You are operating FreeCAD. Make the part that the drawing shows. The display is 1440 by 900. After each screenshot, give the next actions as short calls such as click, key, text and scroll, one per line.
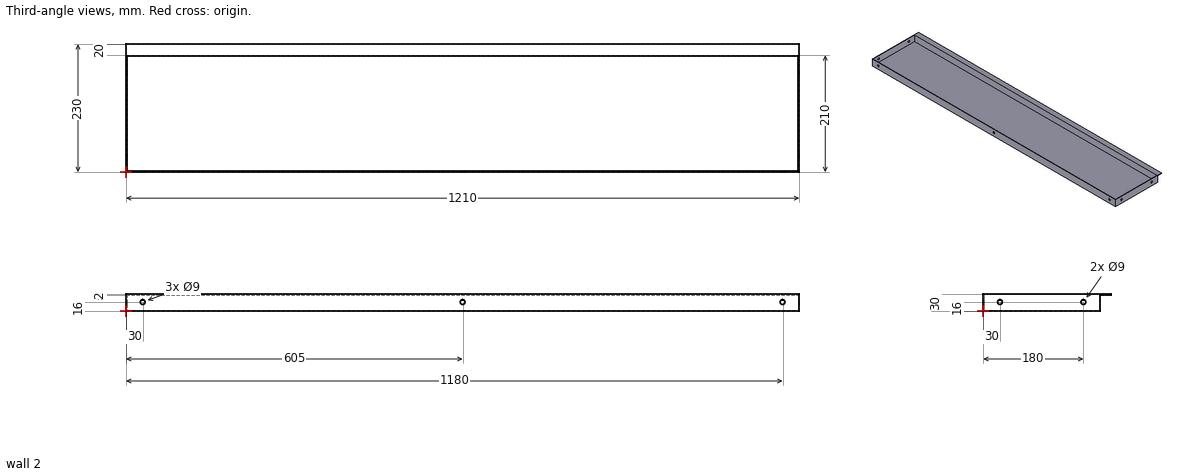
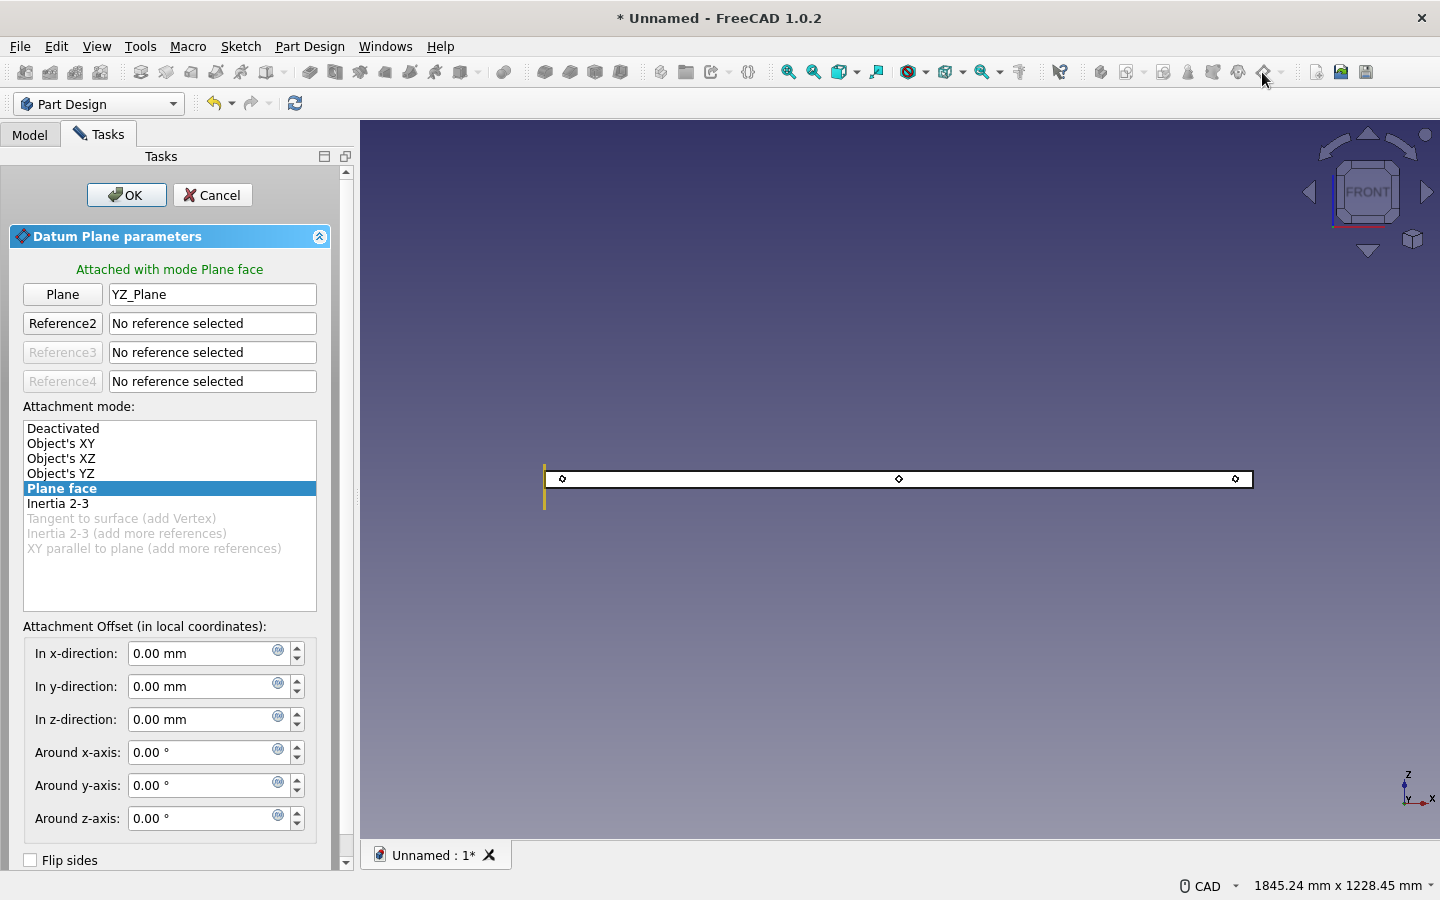
triple_click(210, 720)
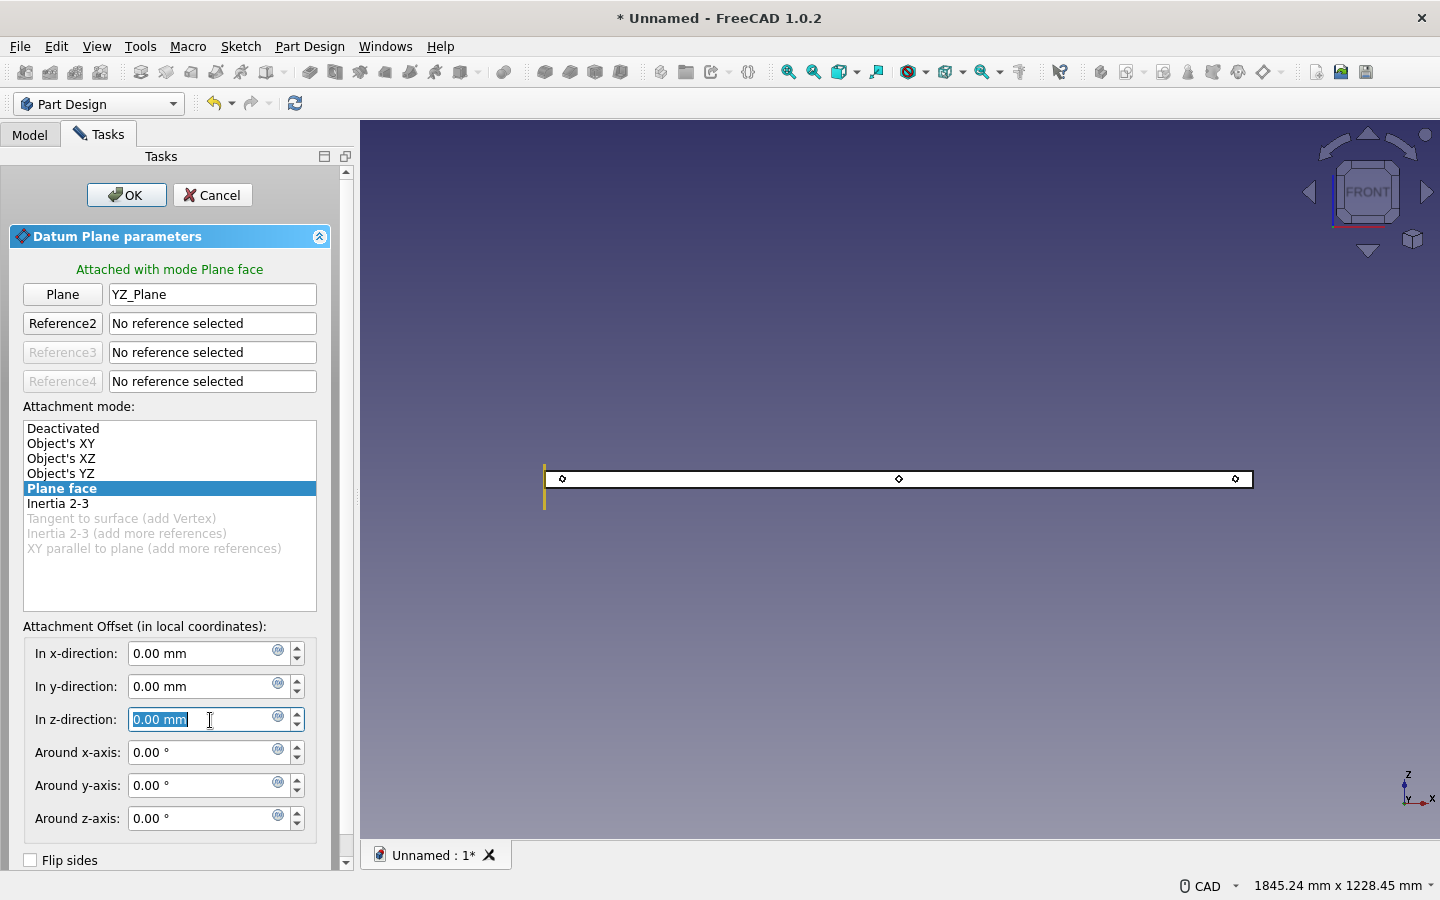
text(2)
key(Tab)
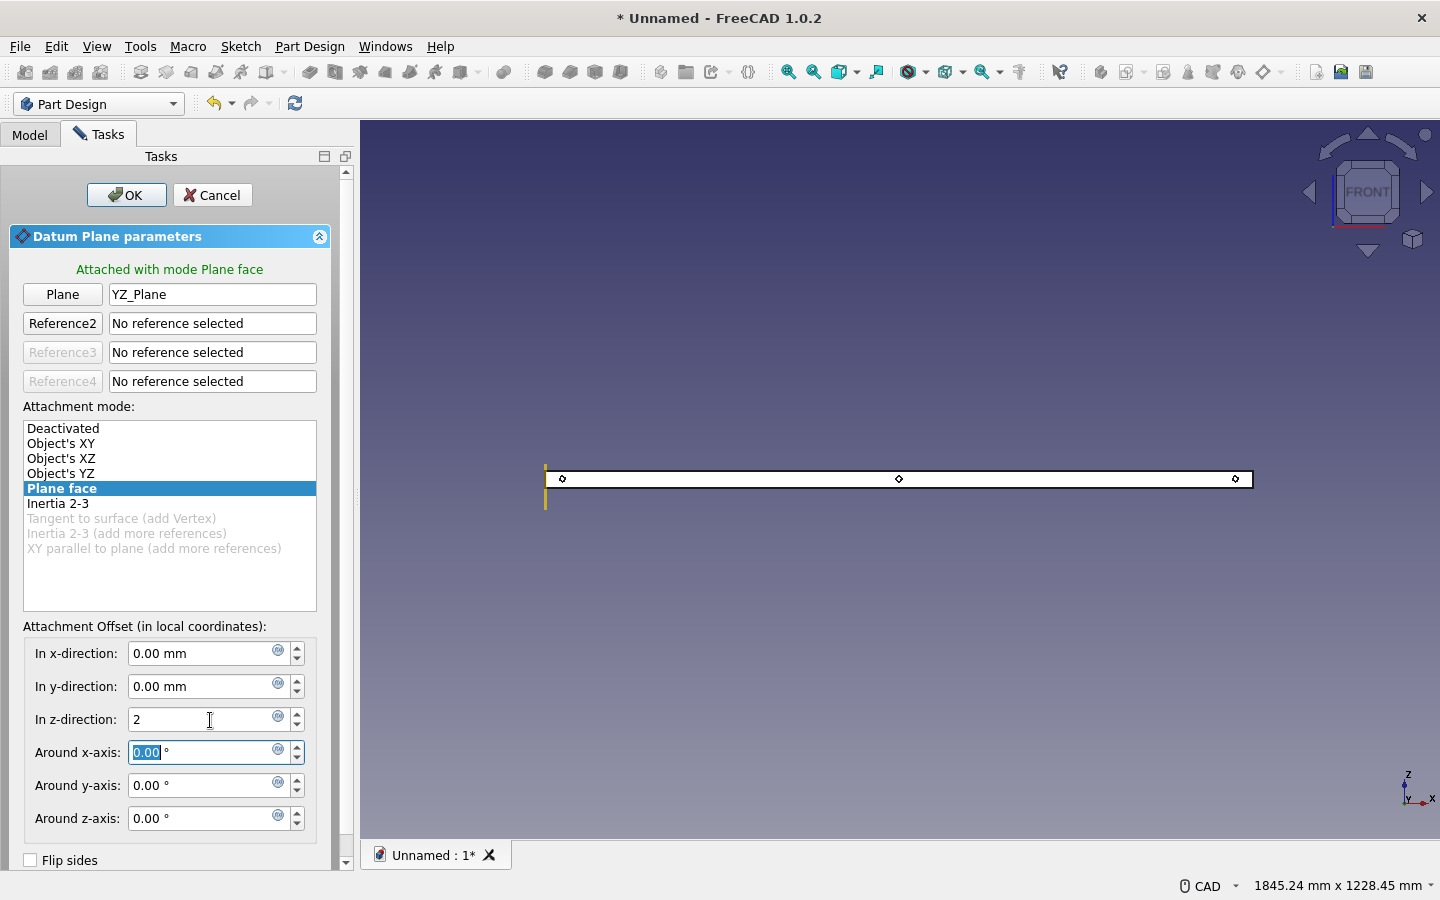
click(127, 195)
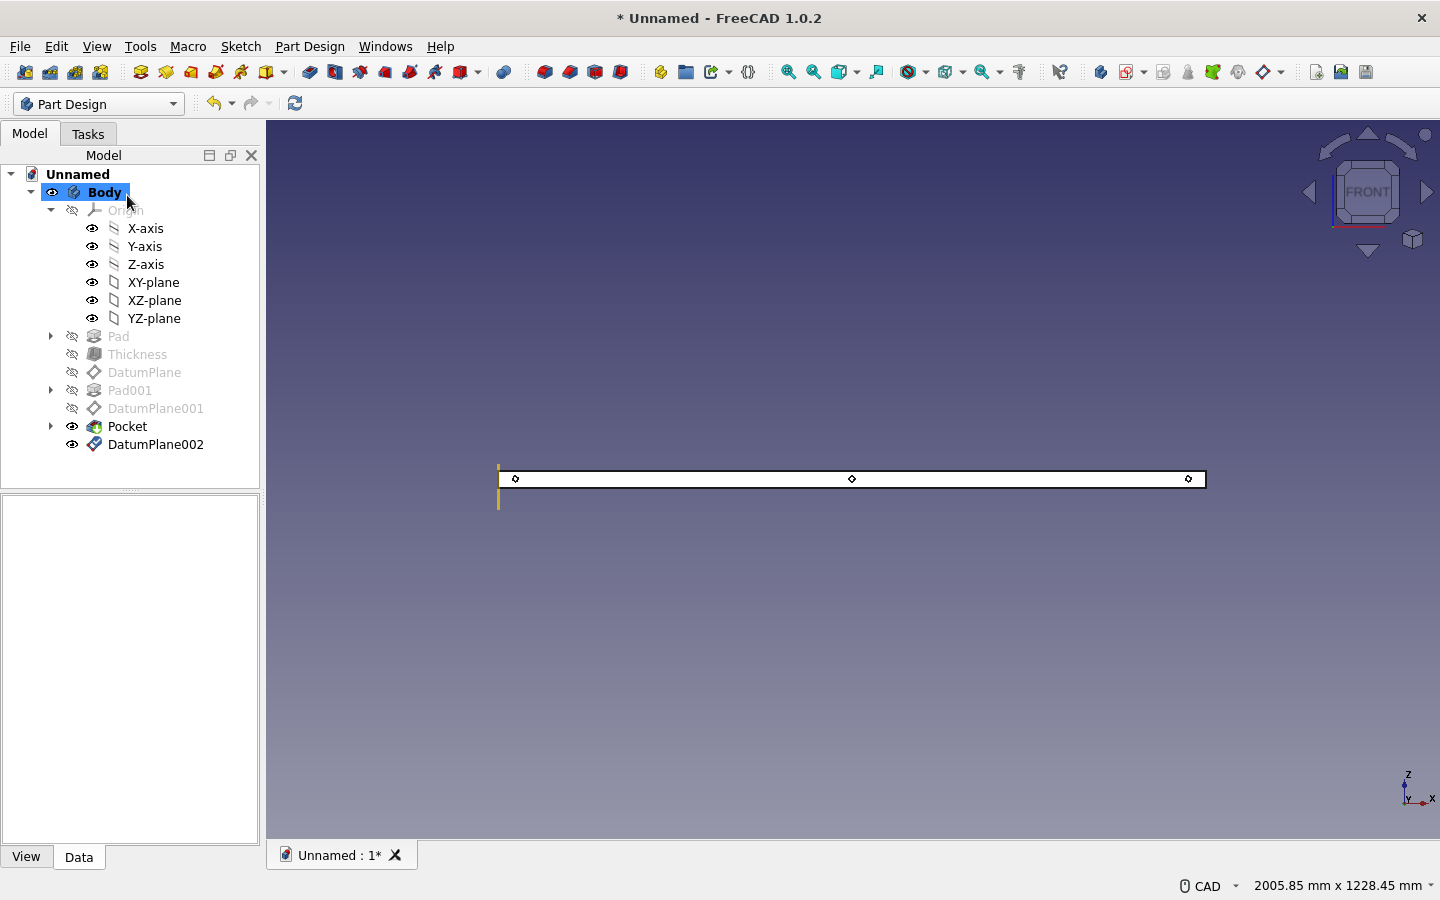
click(117, 444)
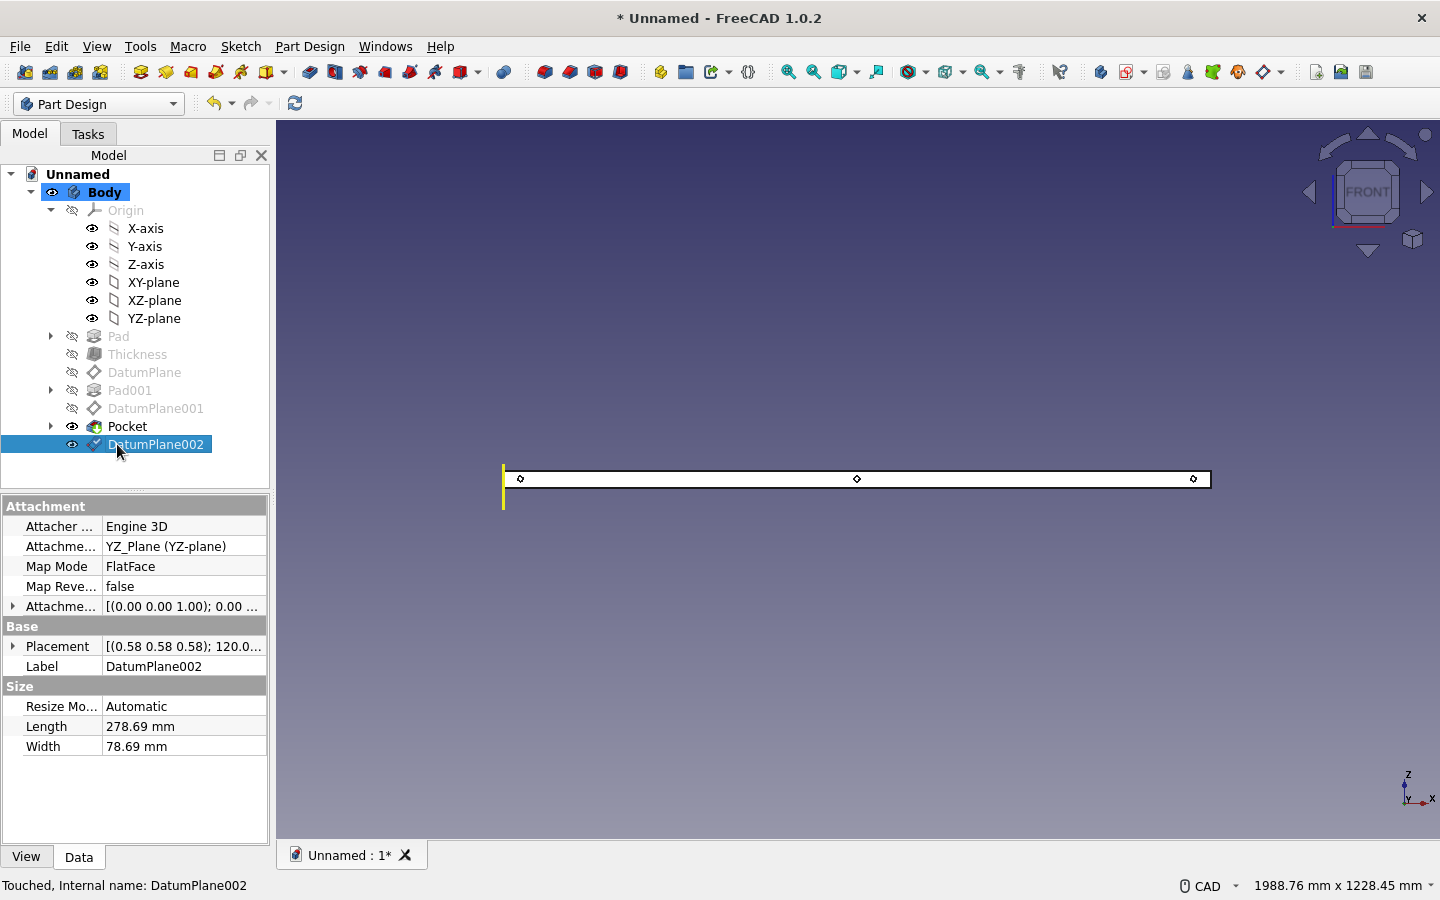
click(1126, 72)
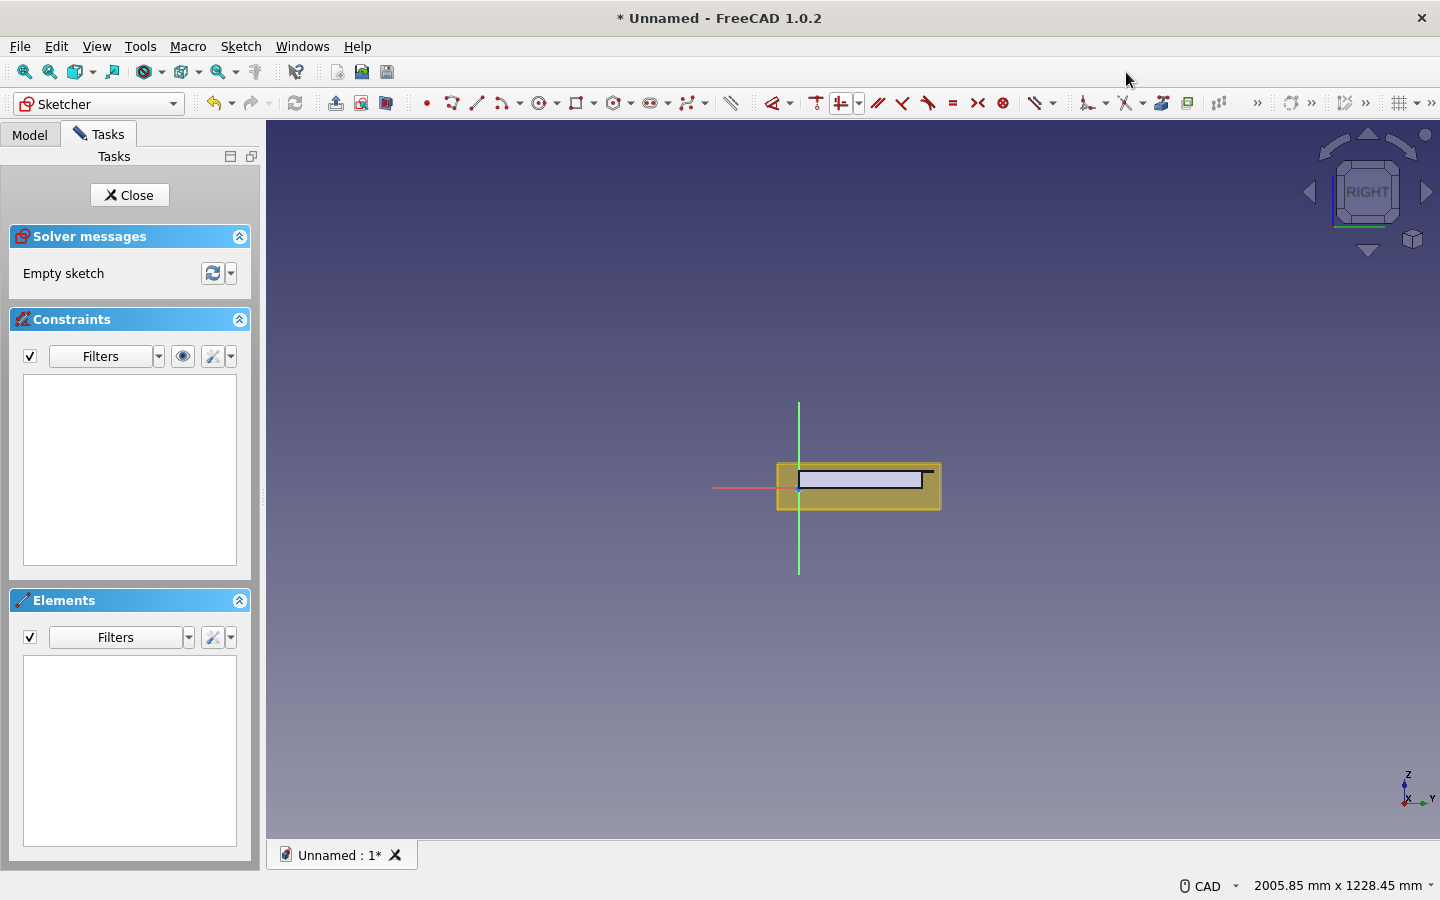
click(386, 104)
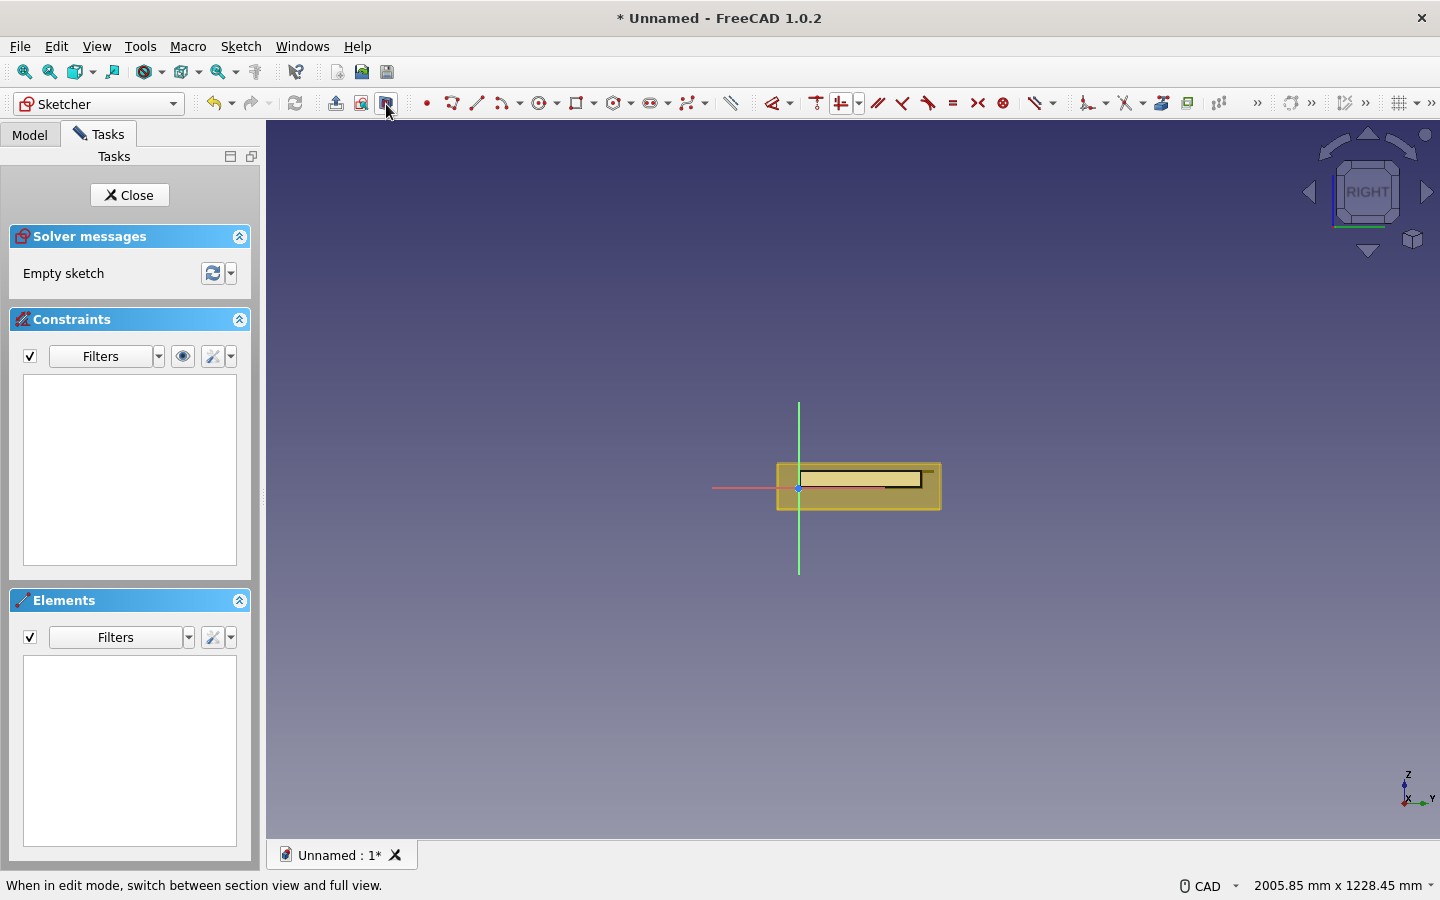
scroll(866, 483, up, 9)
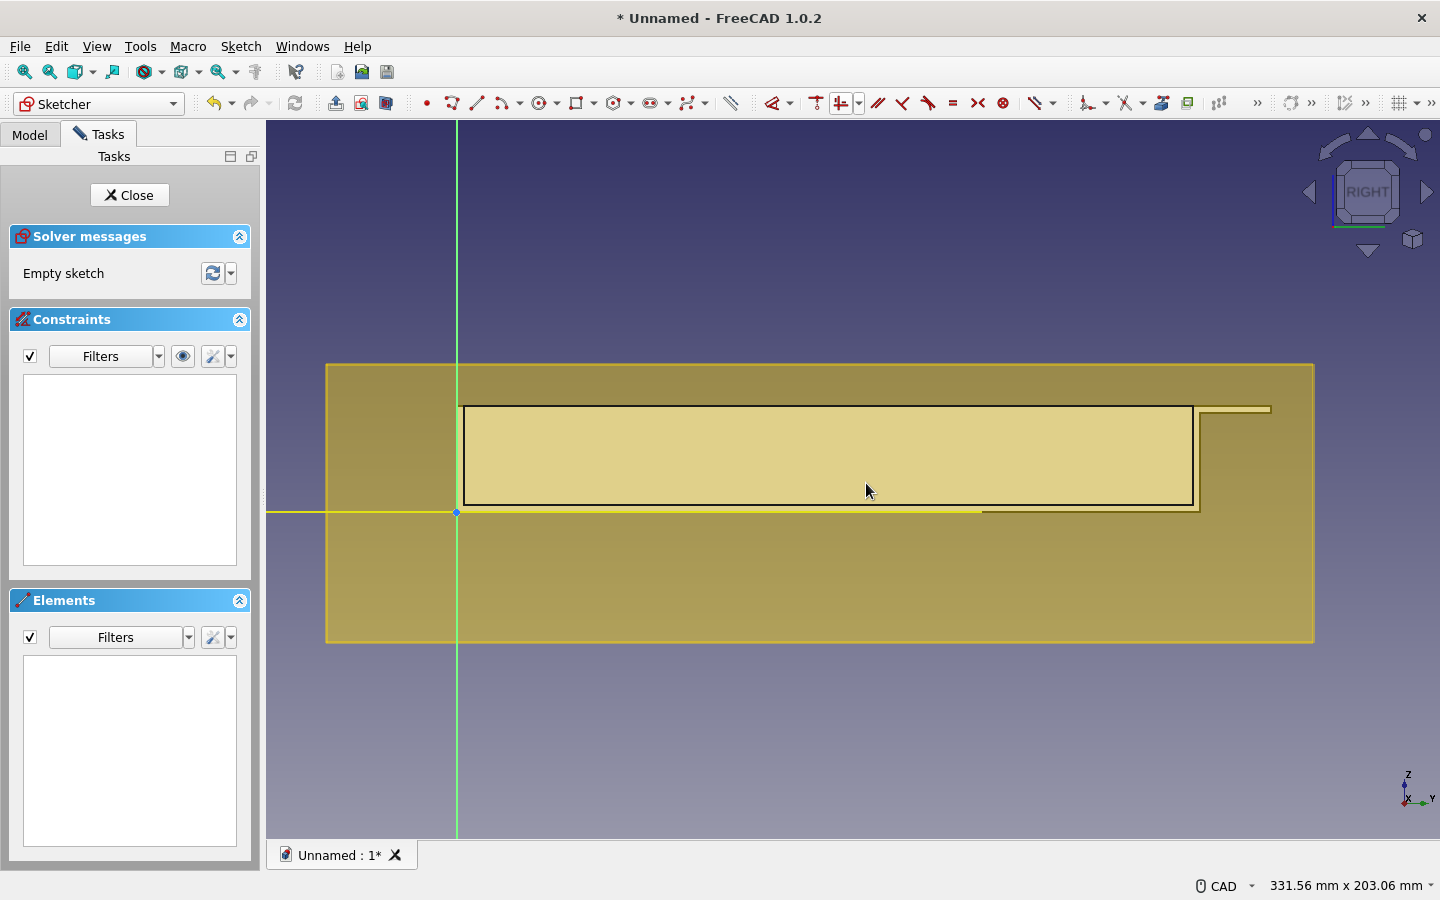
click(538, 104)